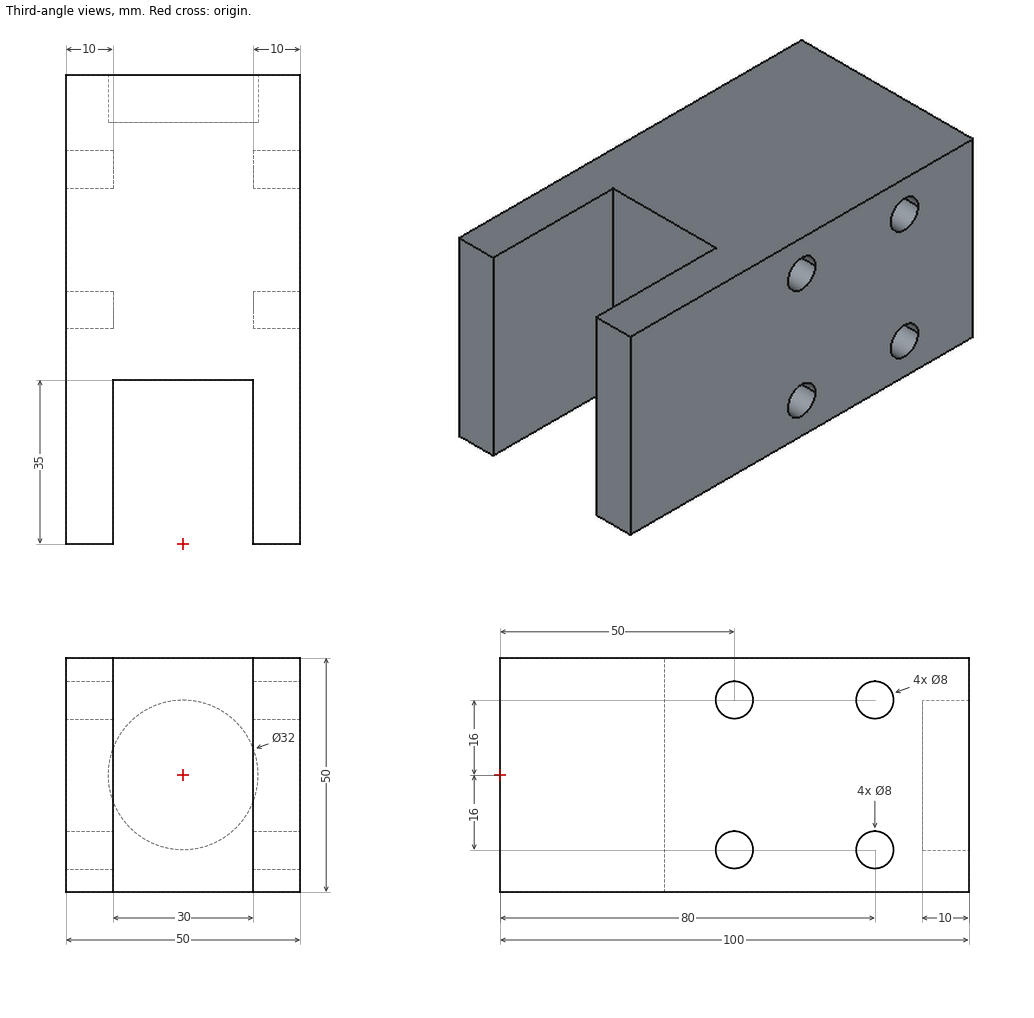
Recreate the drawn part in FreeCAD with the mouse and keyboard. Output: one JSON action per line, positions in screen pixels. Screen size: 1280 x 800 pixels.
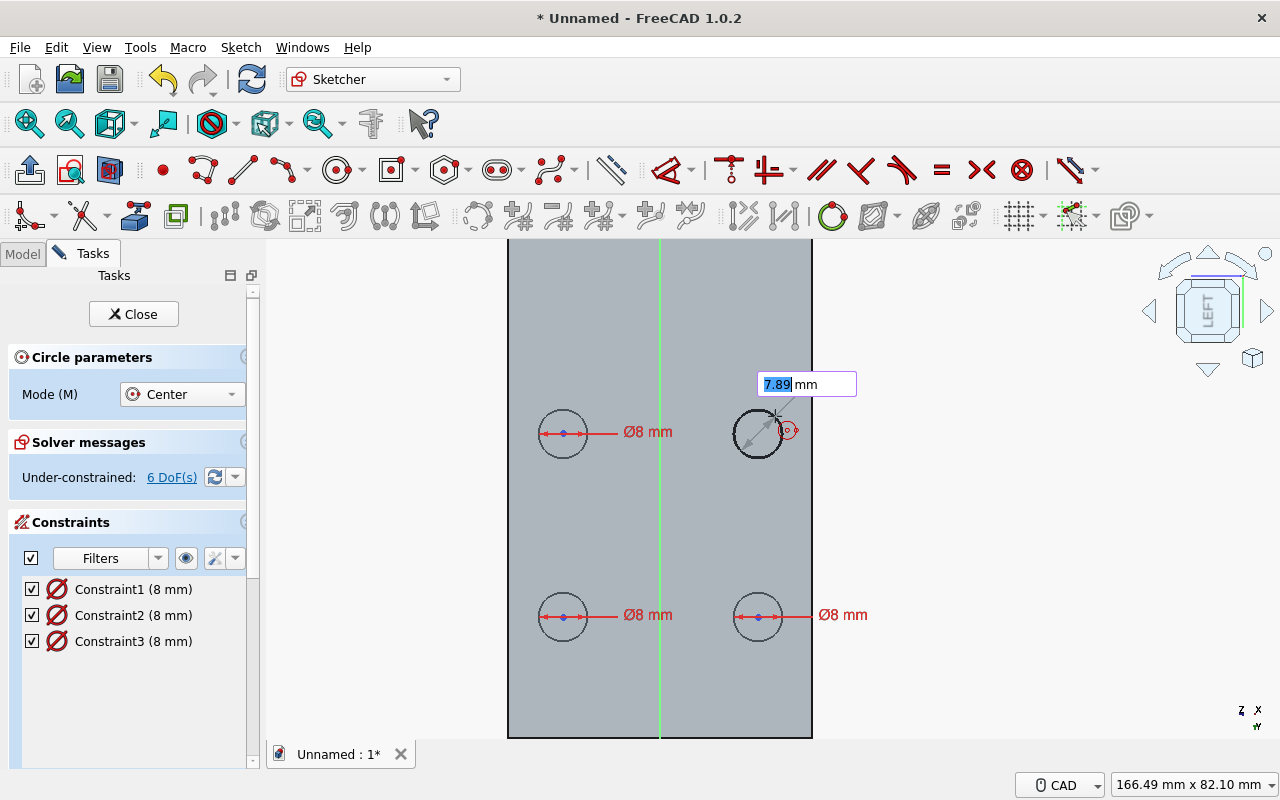
{"action": "type", "text": "8"}
{"action": "key", "text": "Return"}
{"action": "key", "text": "Escape"}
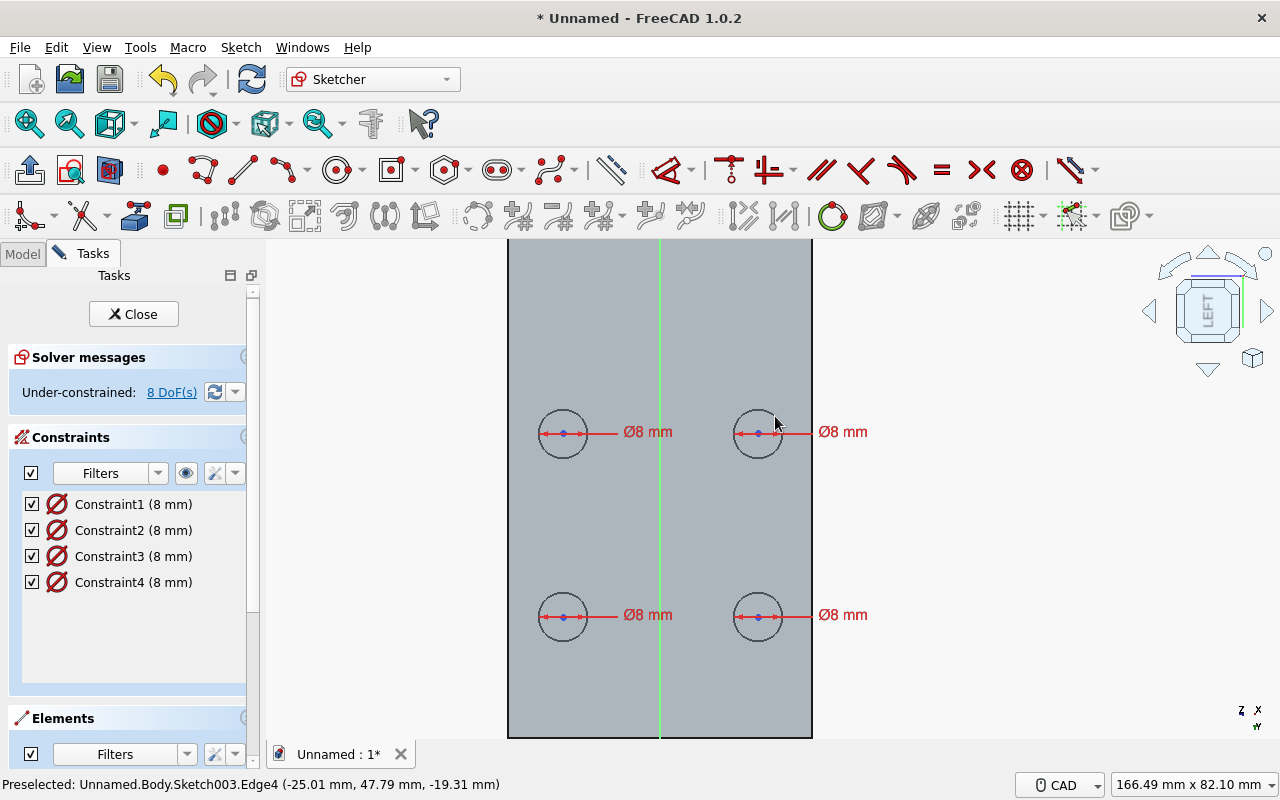
{"action": "left_click", "coordinate": [758, 617]}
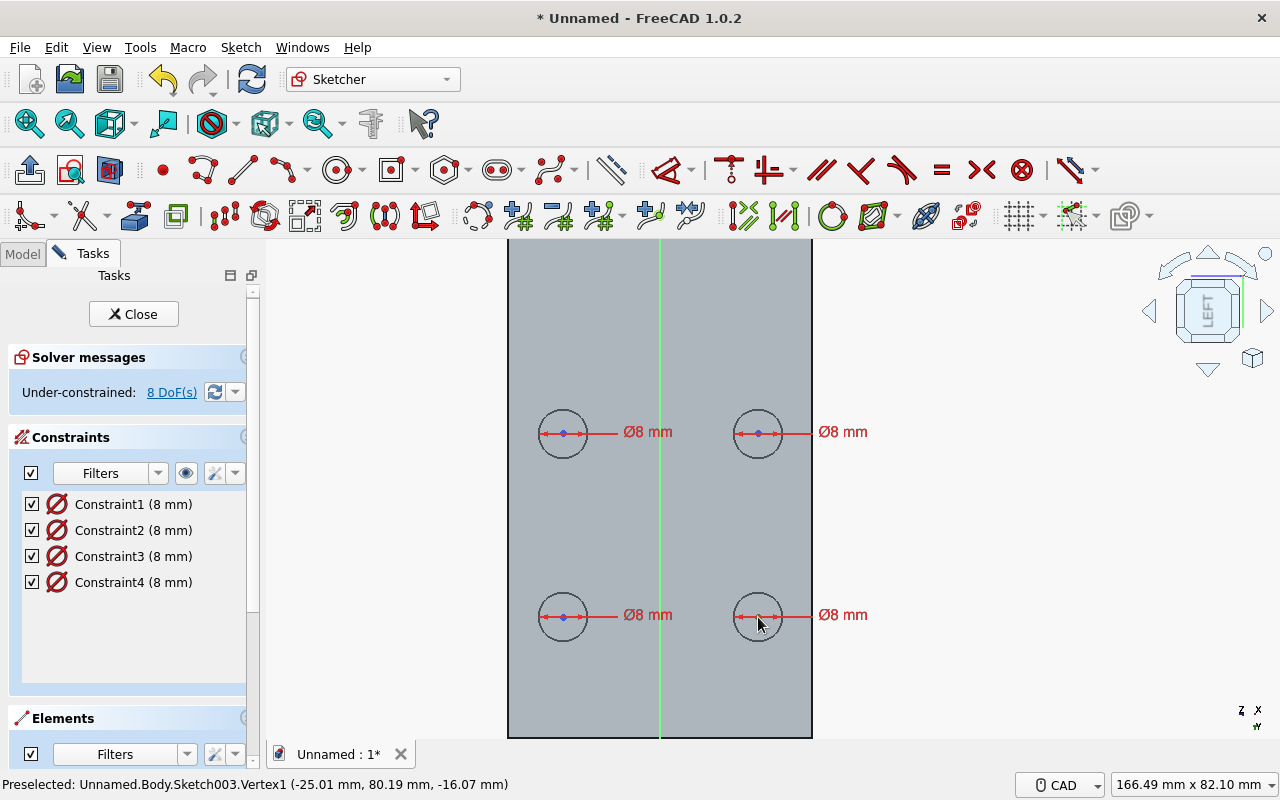
{"action": "left_click", "coordinate": [563, 617]}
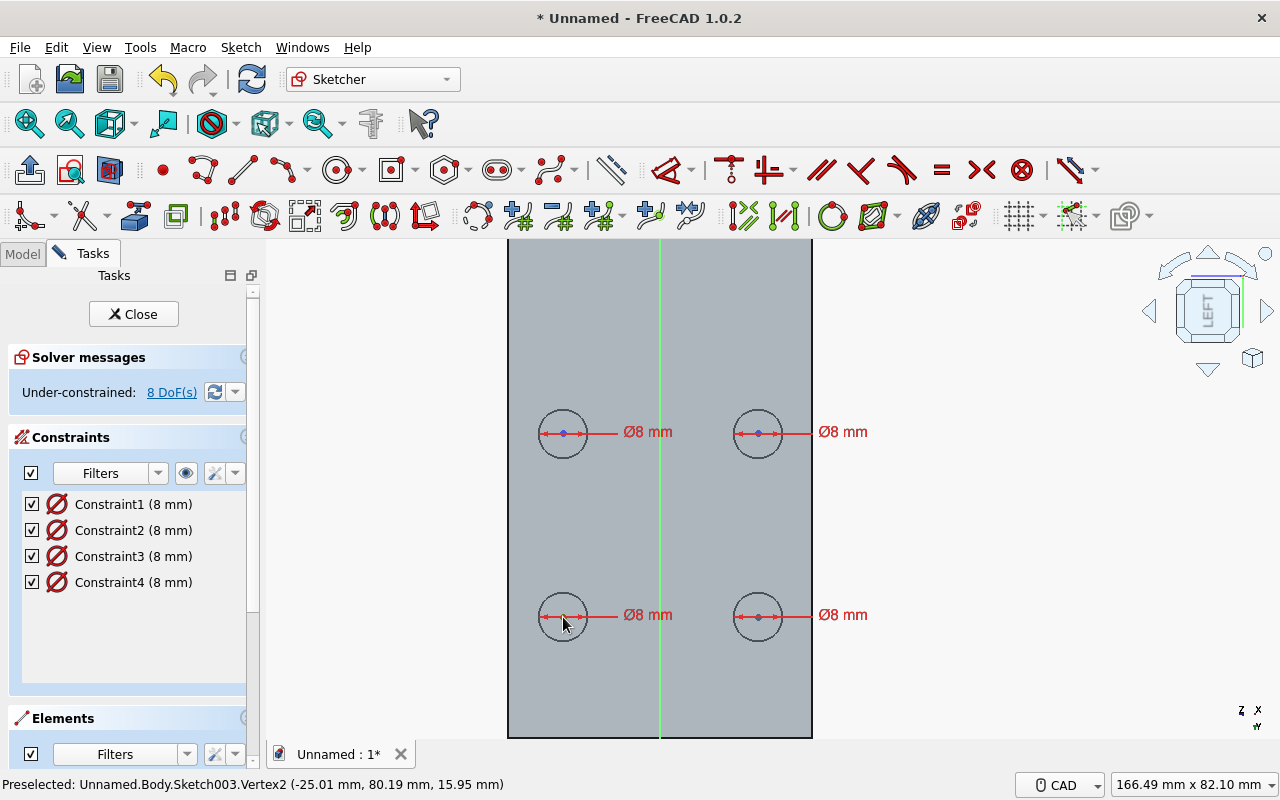
{"action": "key", "text": "h"}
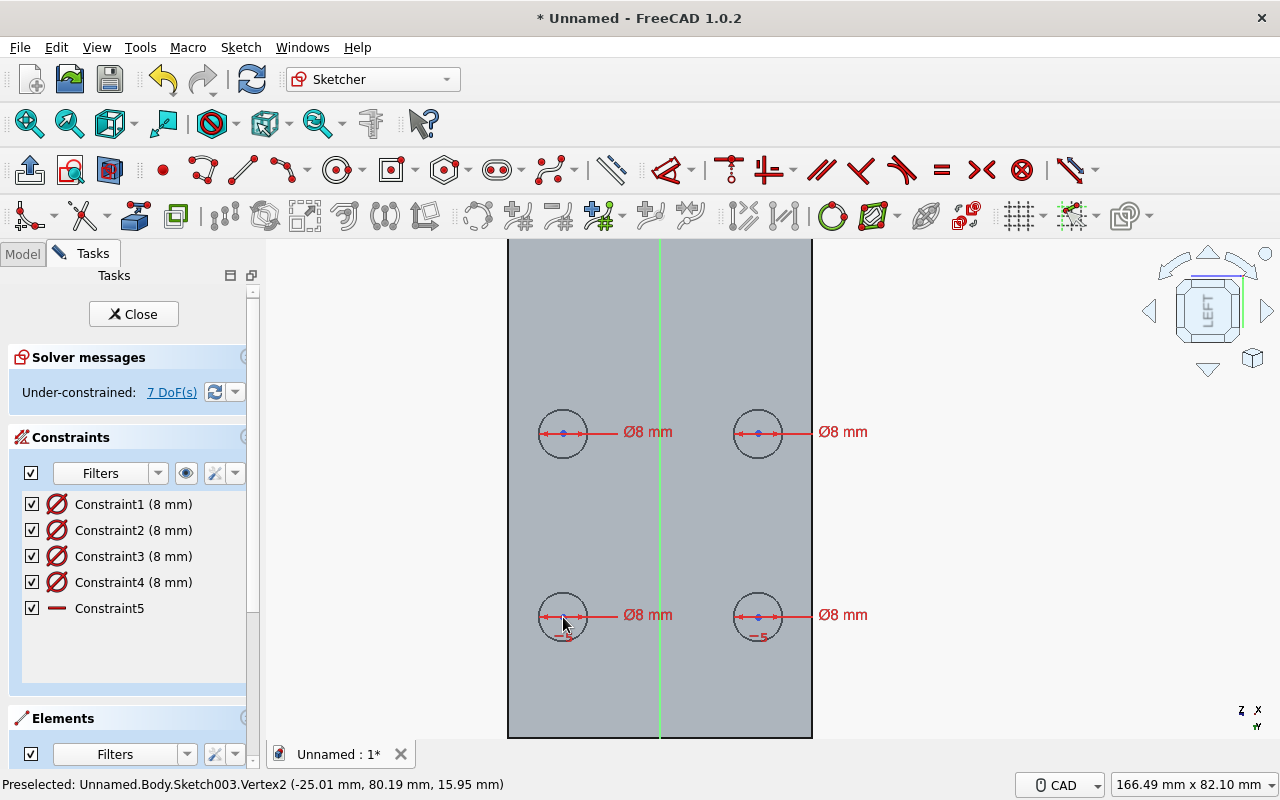
{"action": "left_click", "coordinate": [563, 617]}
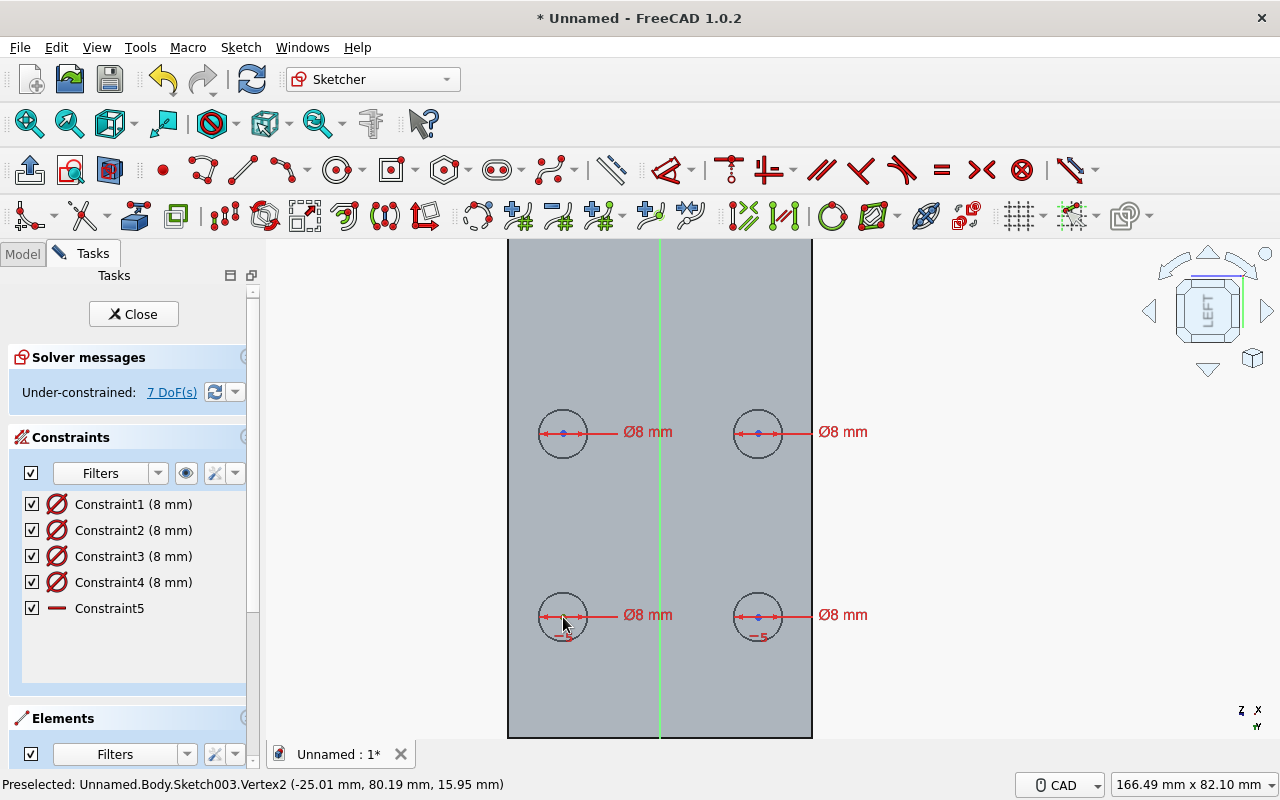
{"action": "left_click", "coordinate": [563, 434]}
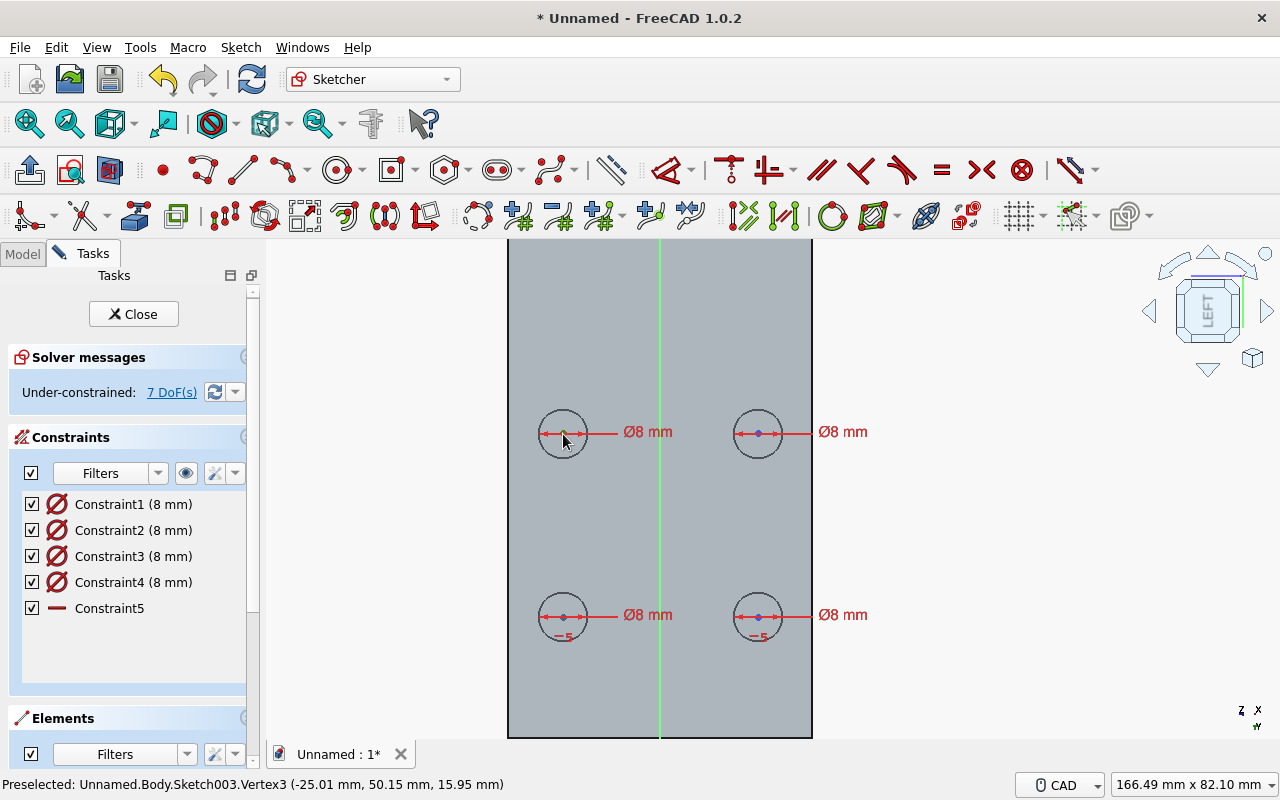
{"action": "left_click", "coordinate": [796, 170]}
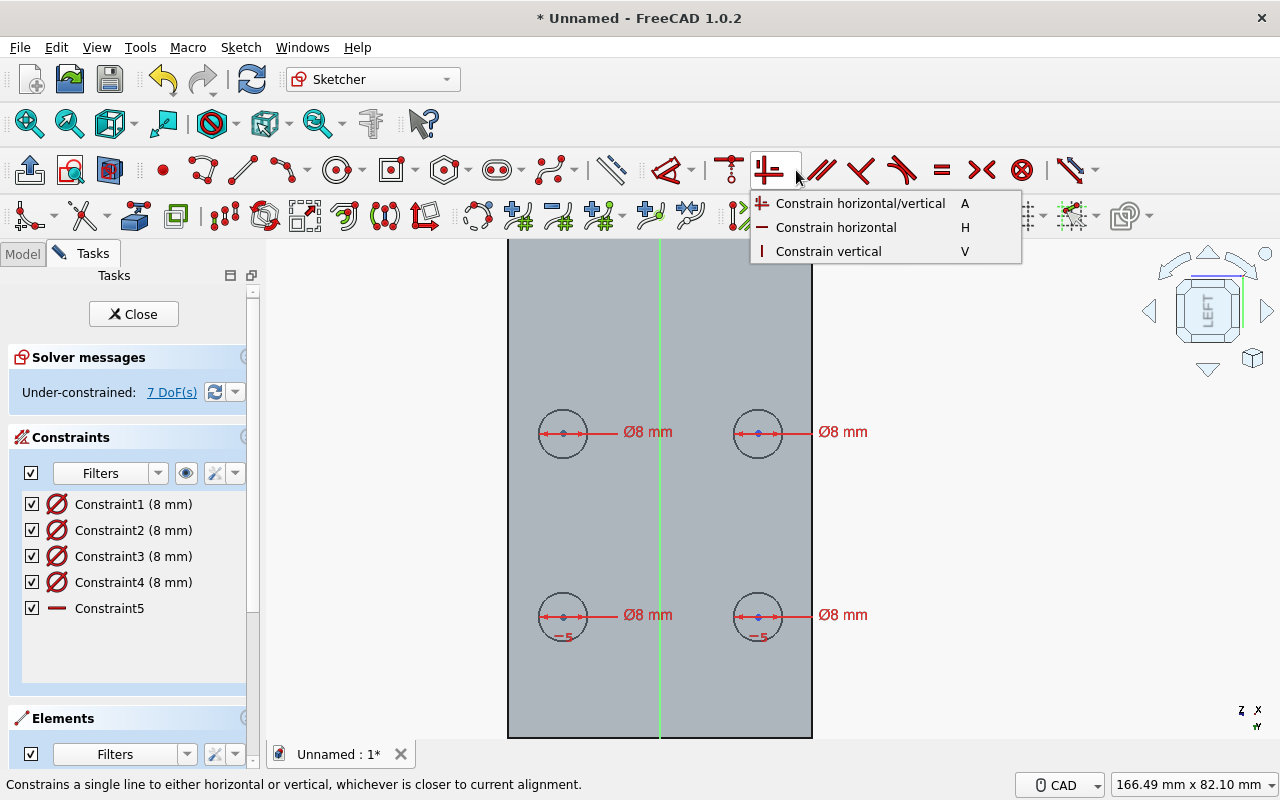
{"action": "left_click", "coordinate": [886, 251]}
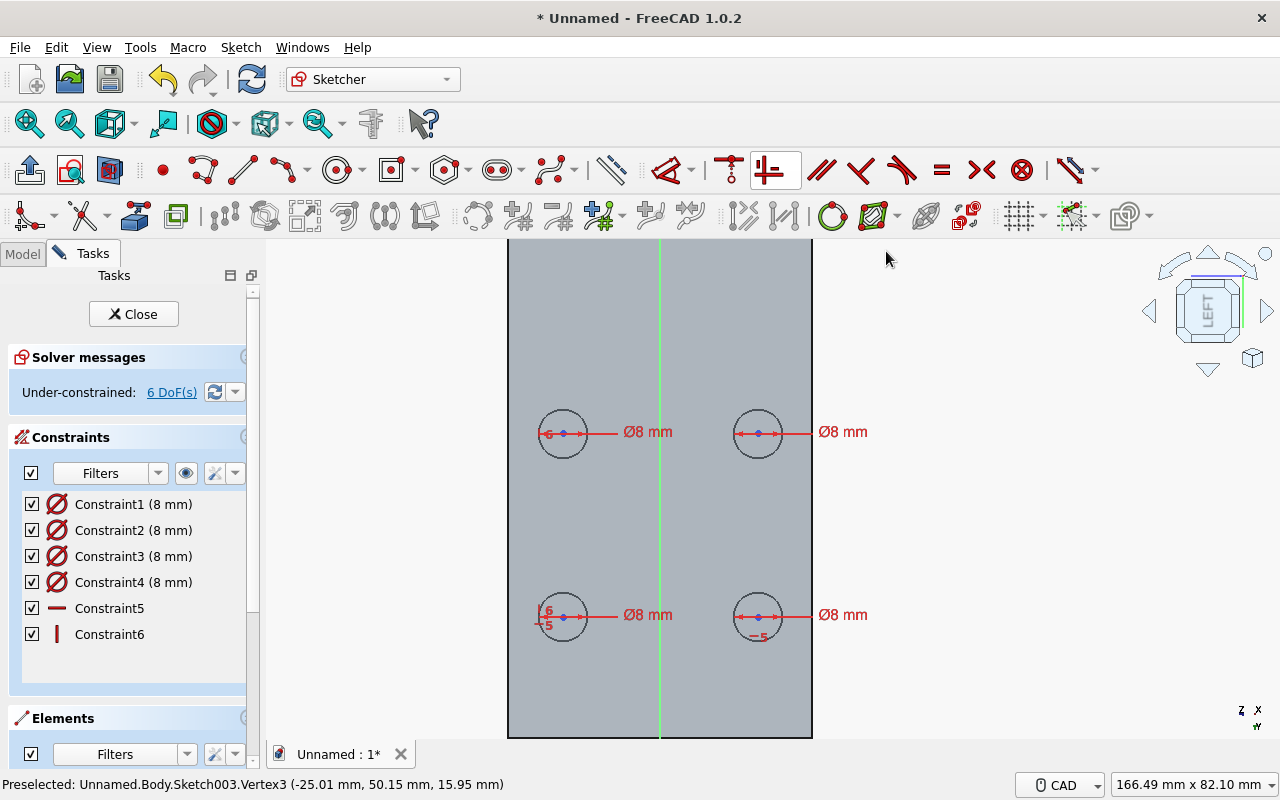
{"action": "left_click", "coordinate": [758, 617]}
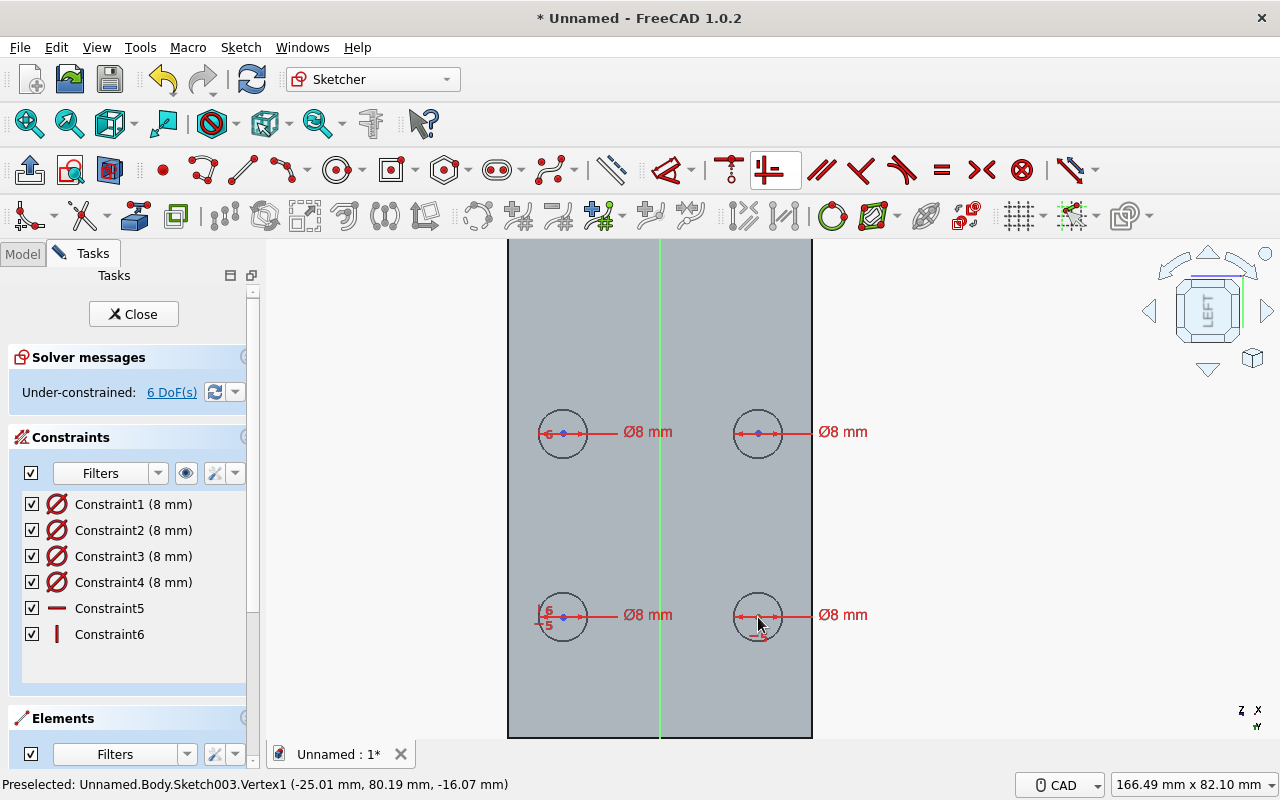
{"action": "left_click", "coordinate": [758, 434]}